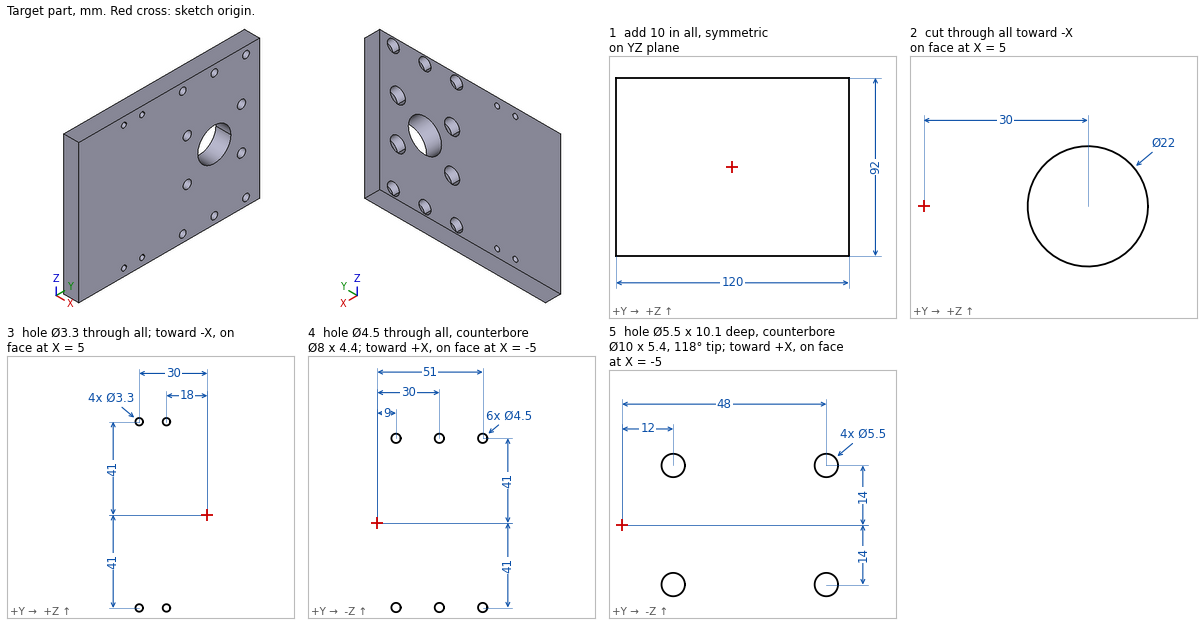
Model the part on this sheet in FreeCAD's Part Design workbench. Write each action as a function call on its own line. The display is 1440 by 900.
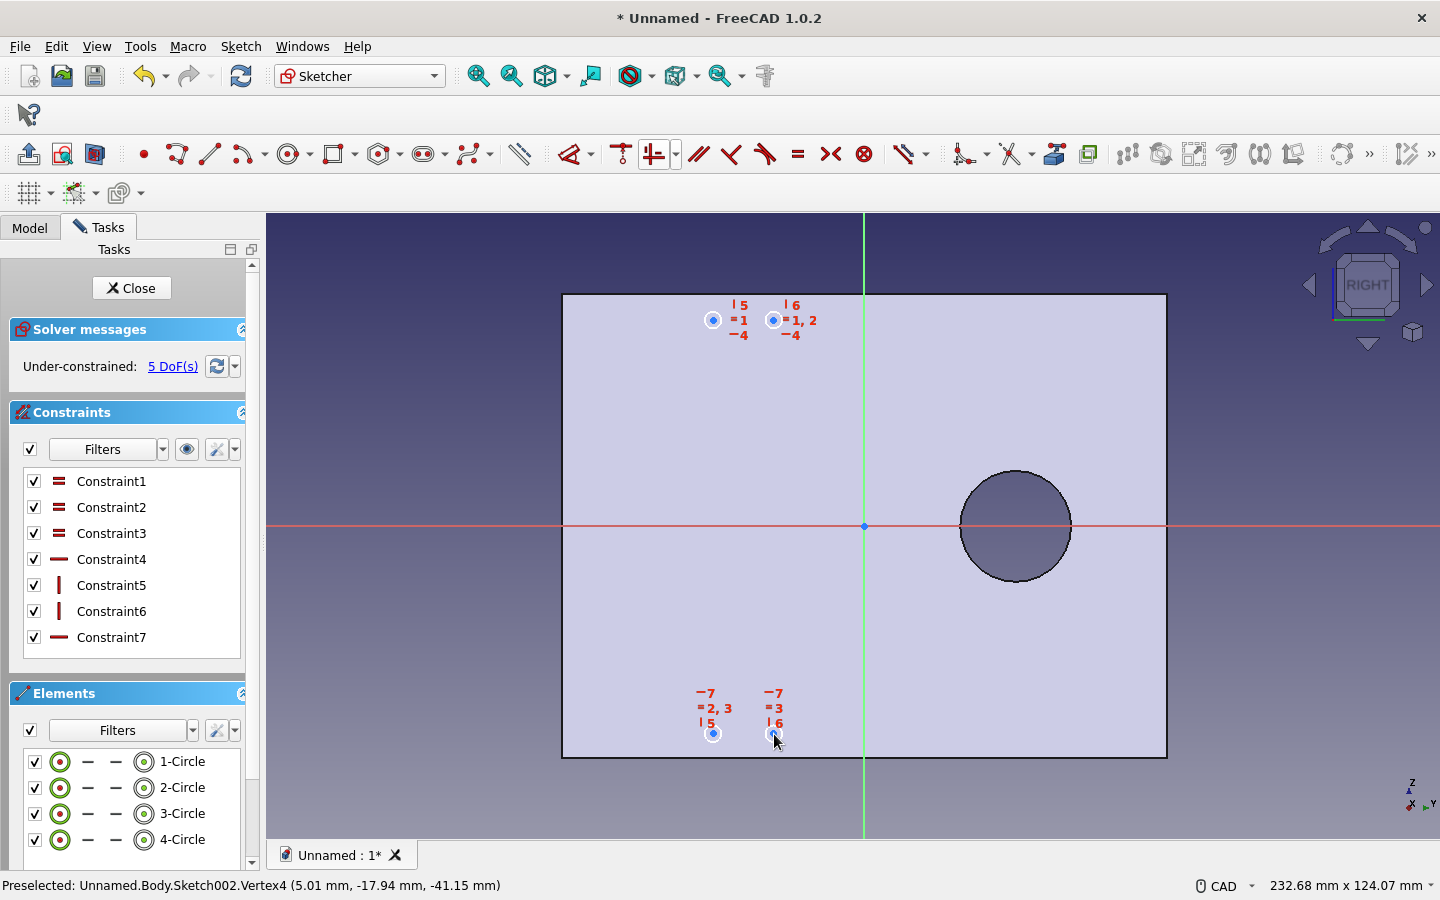
key(d)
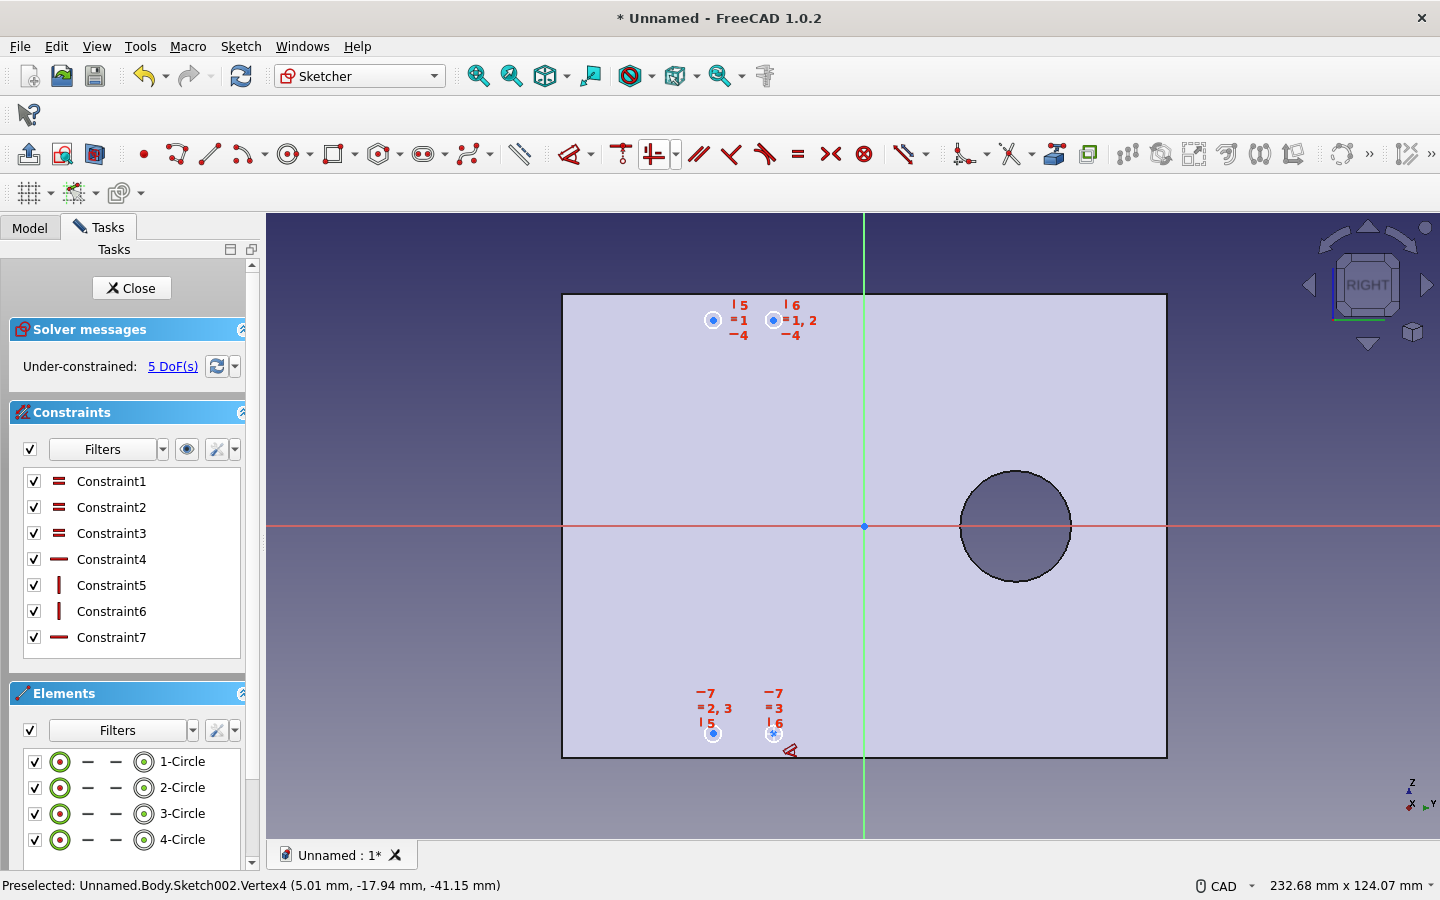
scroll(719, 314, up, 5)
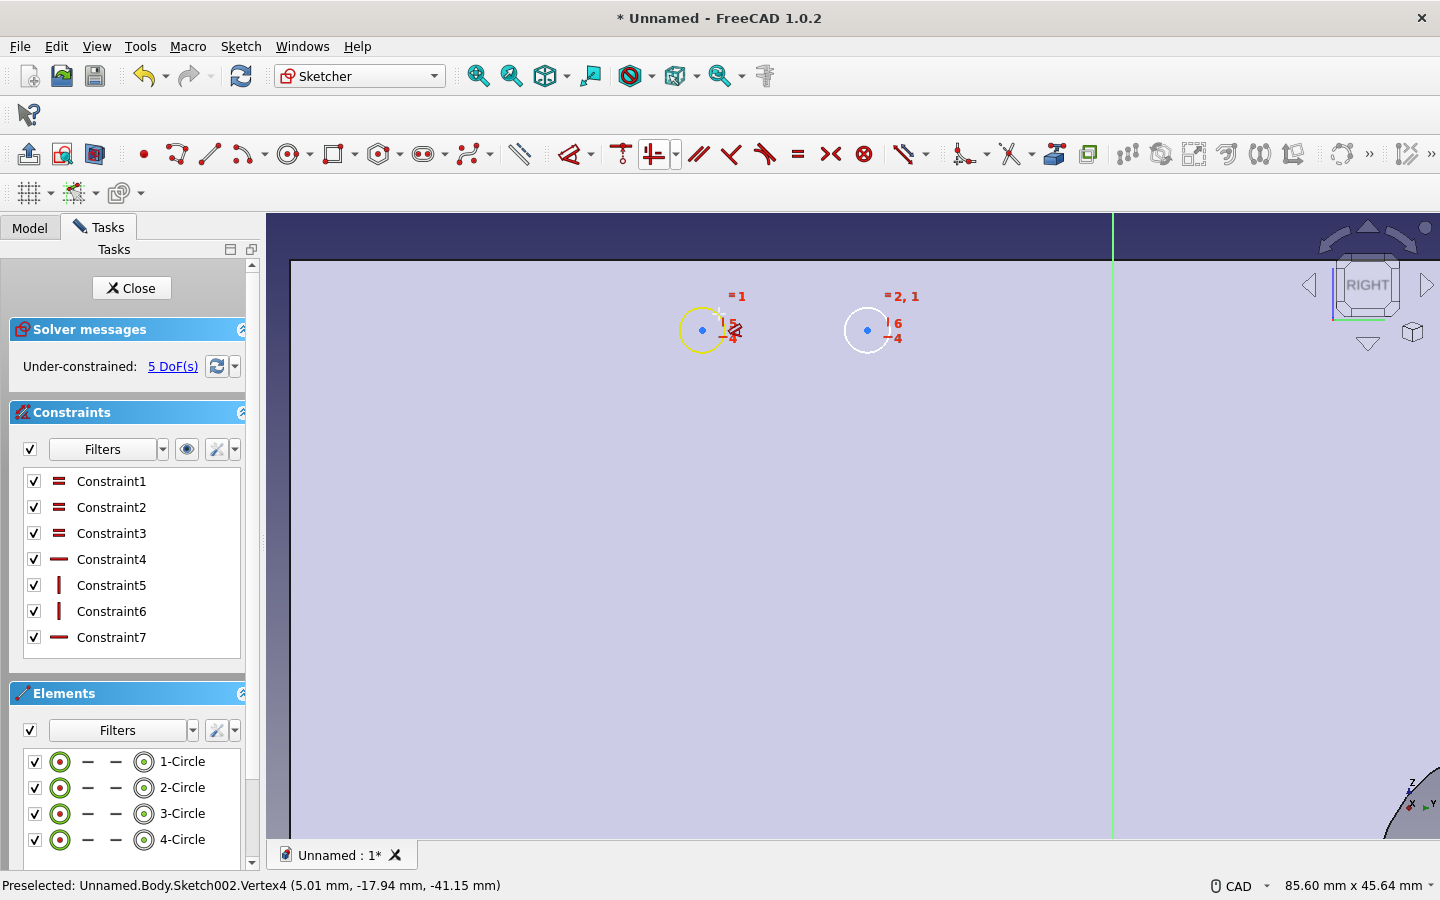
click(718, 314)
click(740, 291)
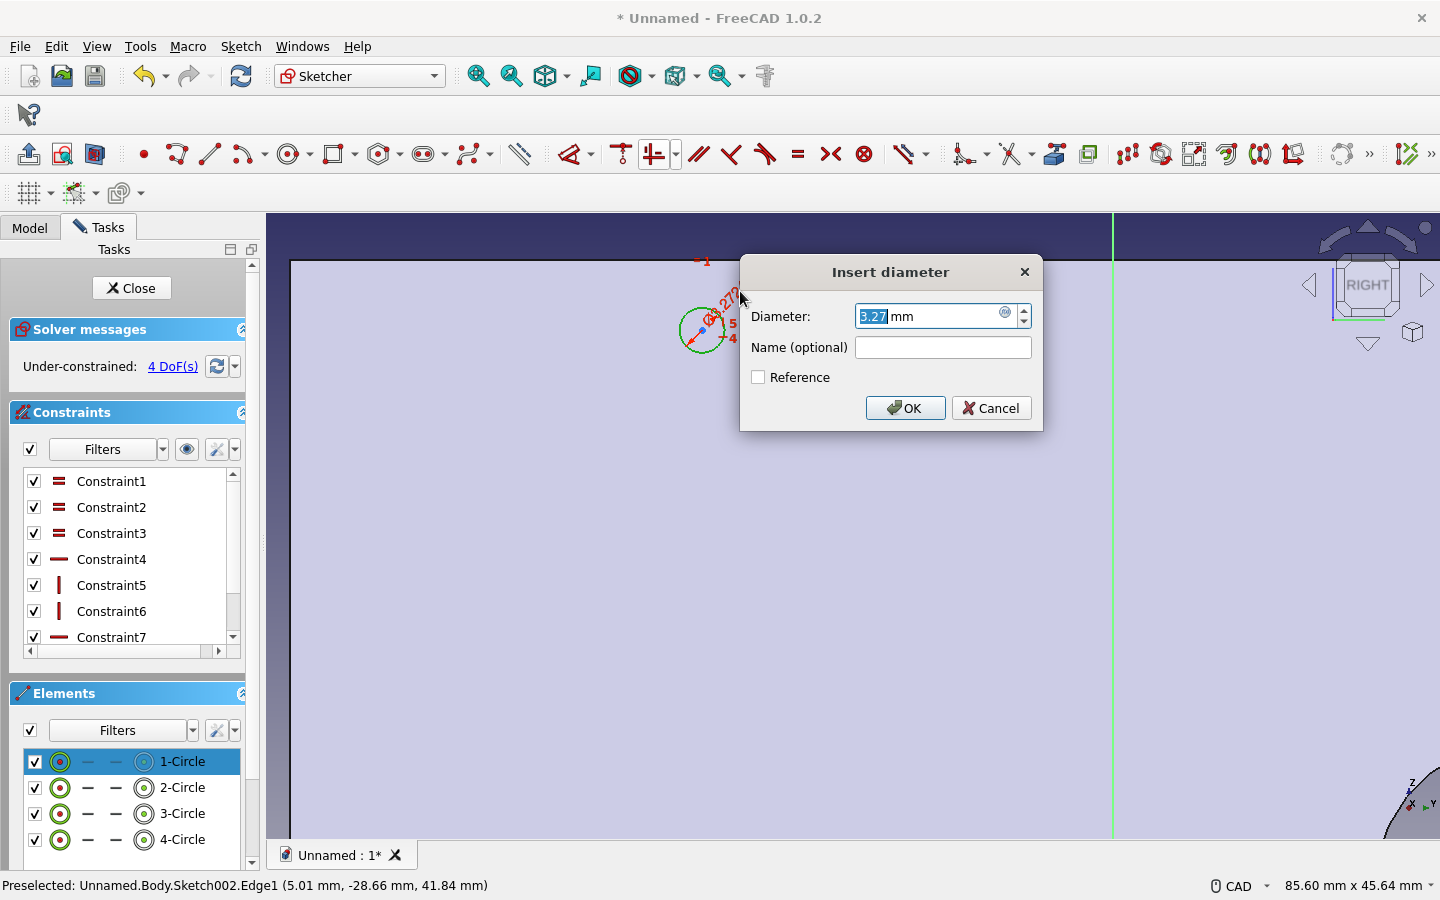
text(3.3)
key(Return)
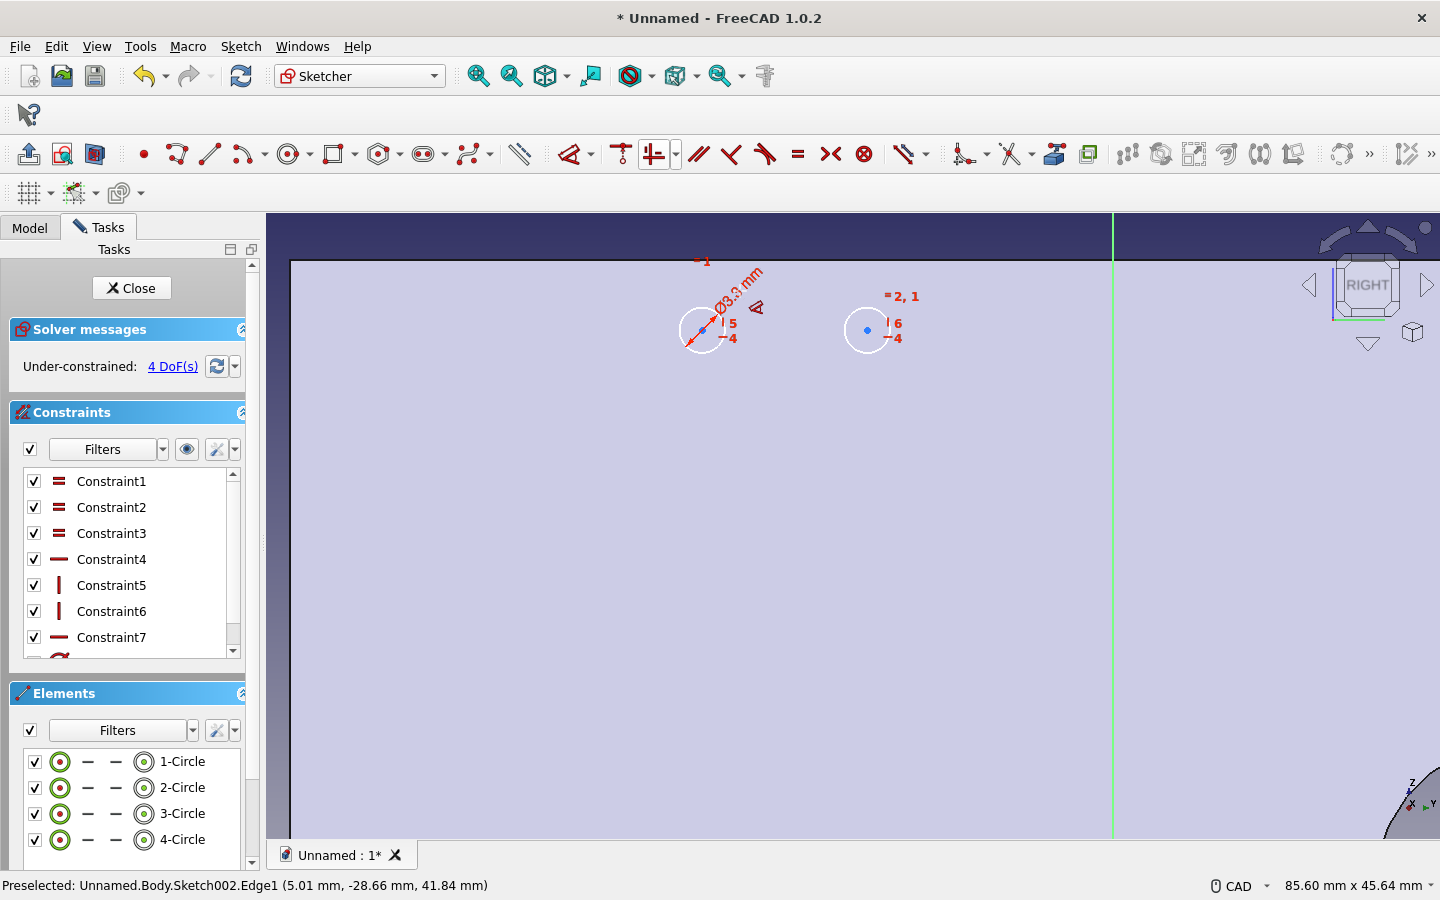
click(702, 330)
click(908, 296)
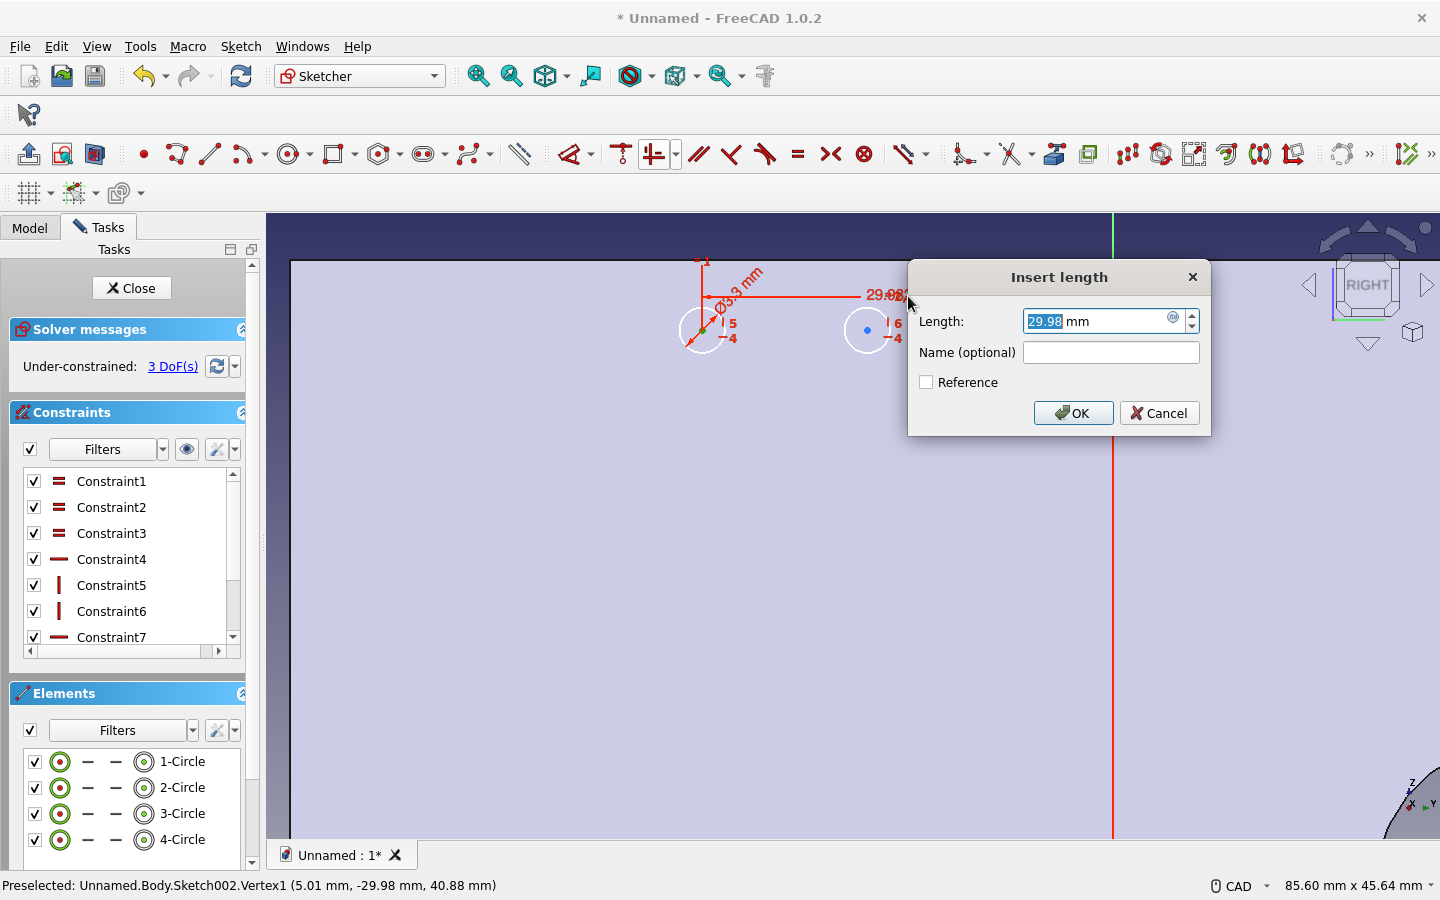
text(30)
key(Return)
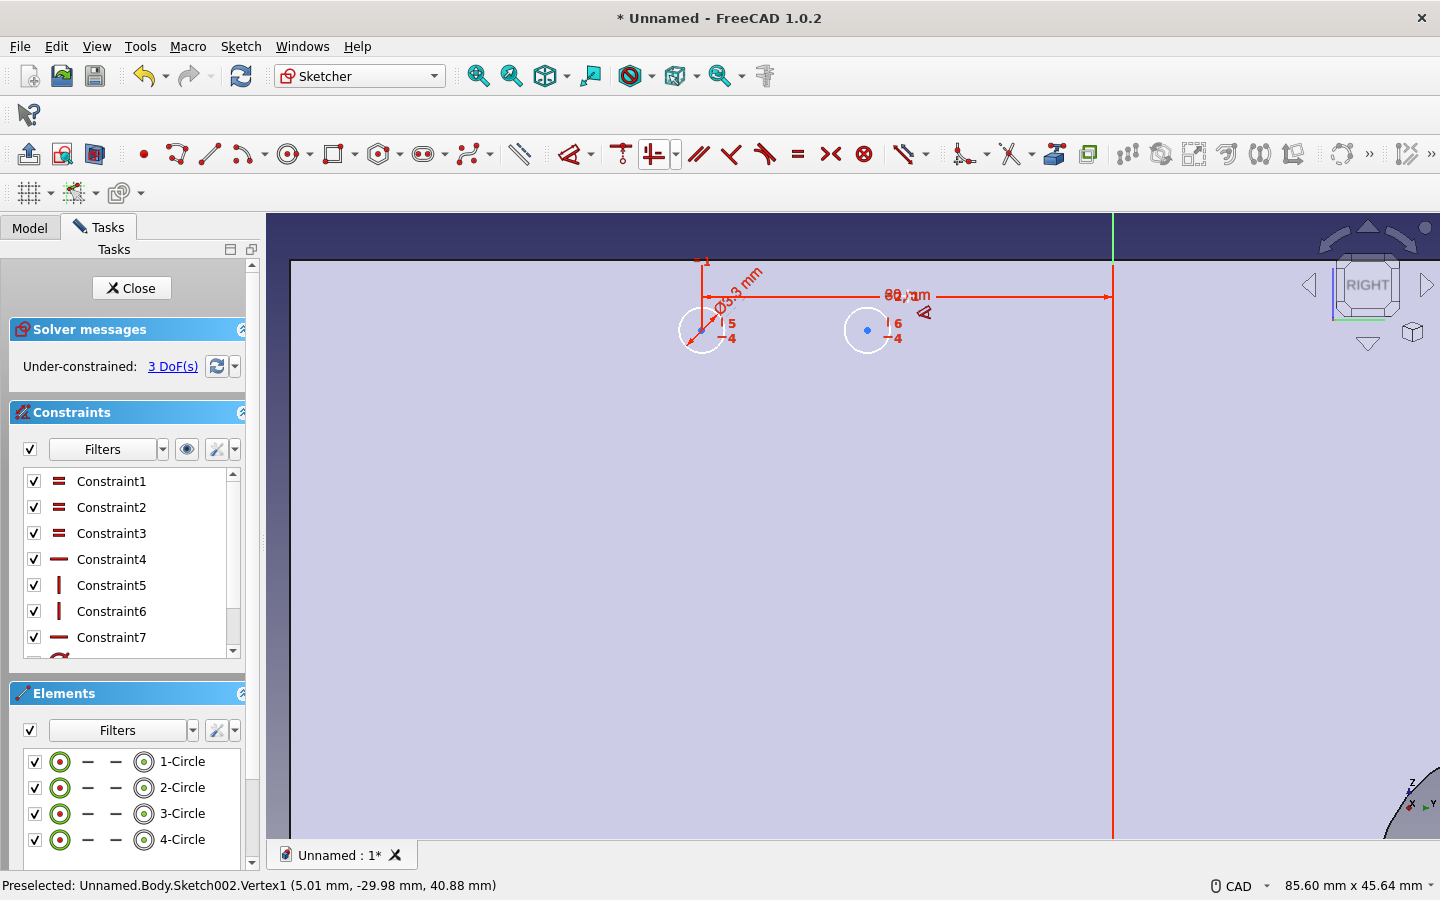
click(702, 330)
click(1147, 571)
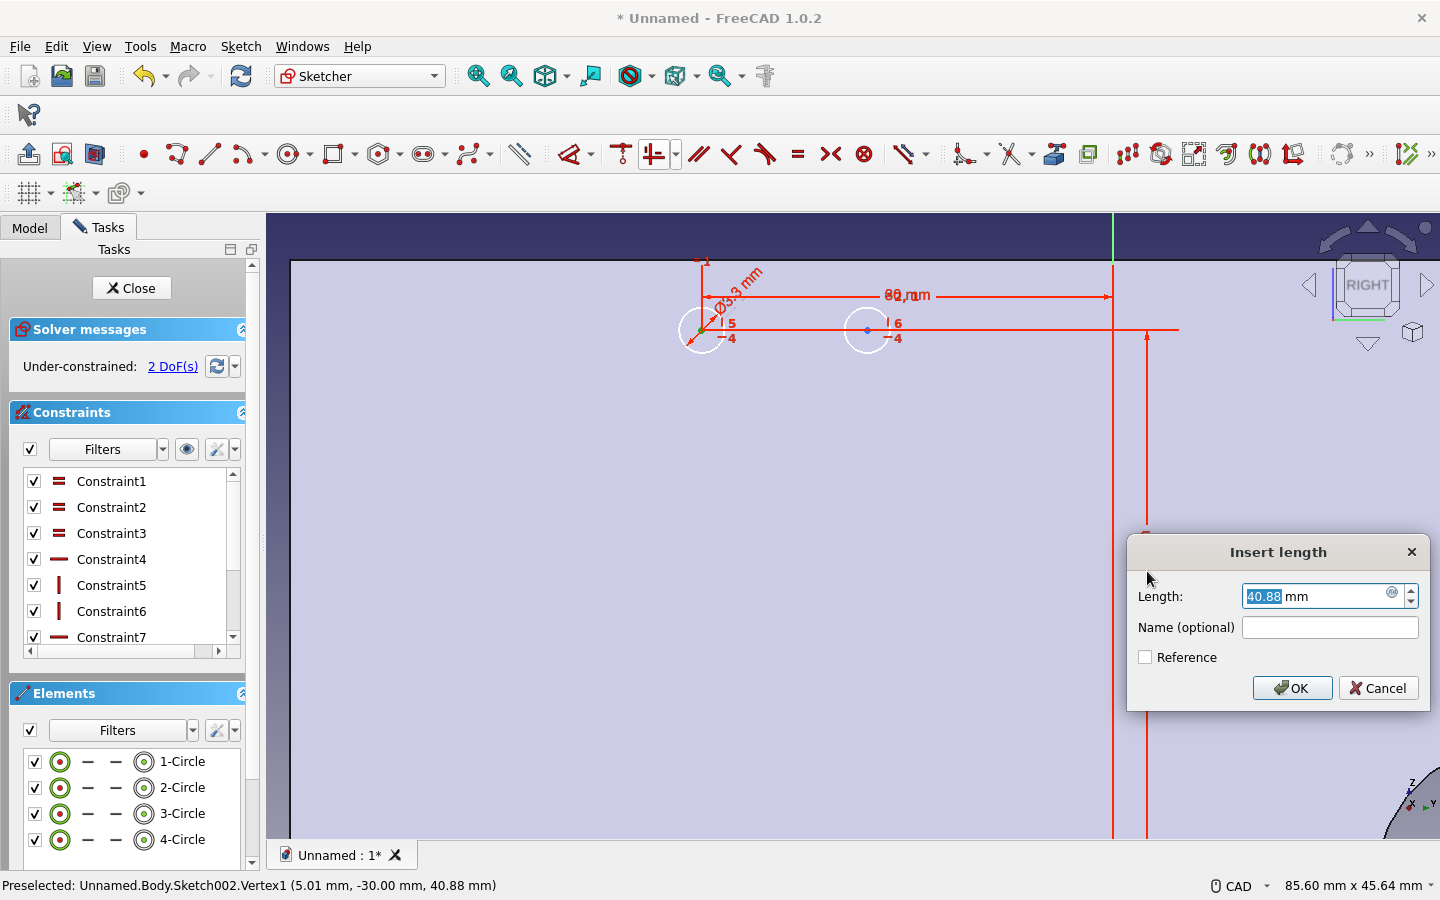
text(41)
key(Return)